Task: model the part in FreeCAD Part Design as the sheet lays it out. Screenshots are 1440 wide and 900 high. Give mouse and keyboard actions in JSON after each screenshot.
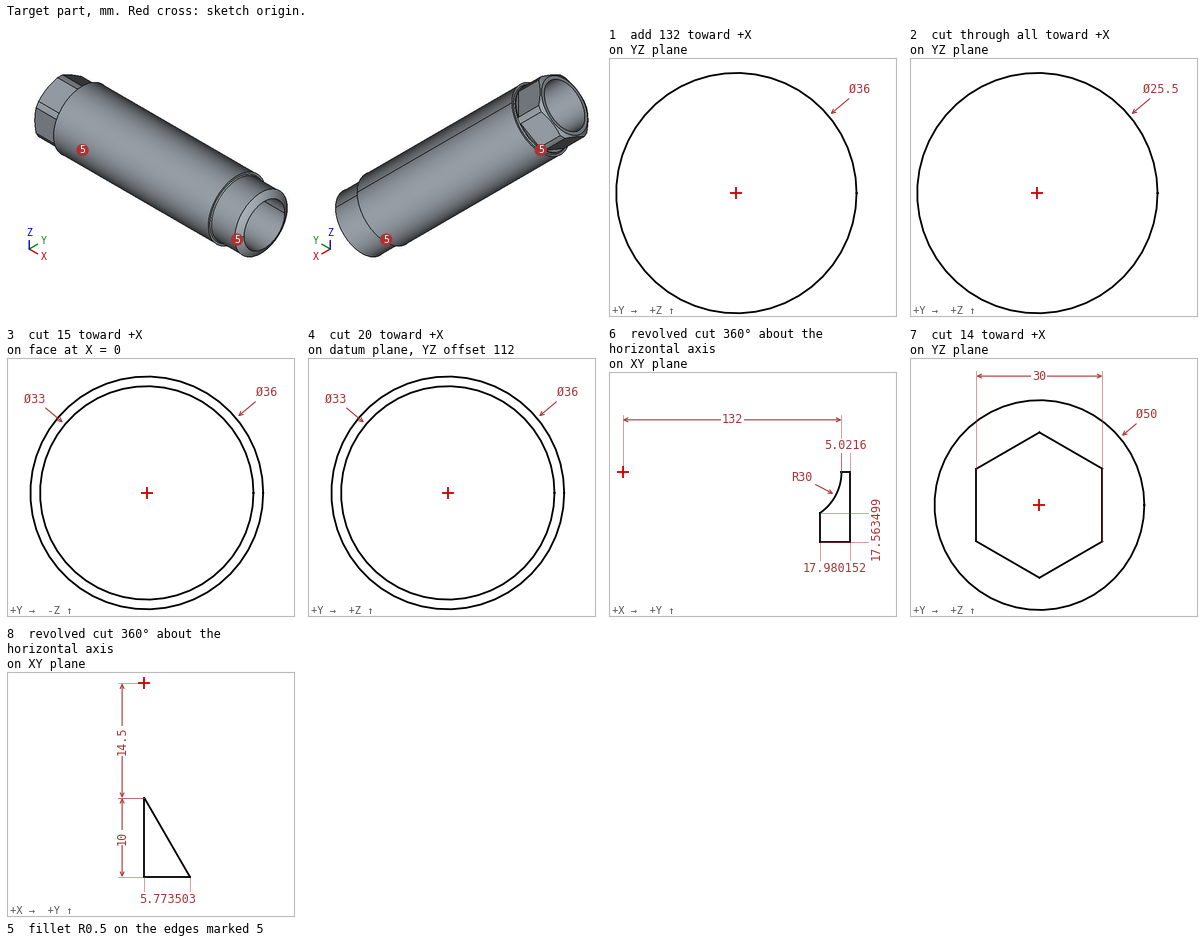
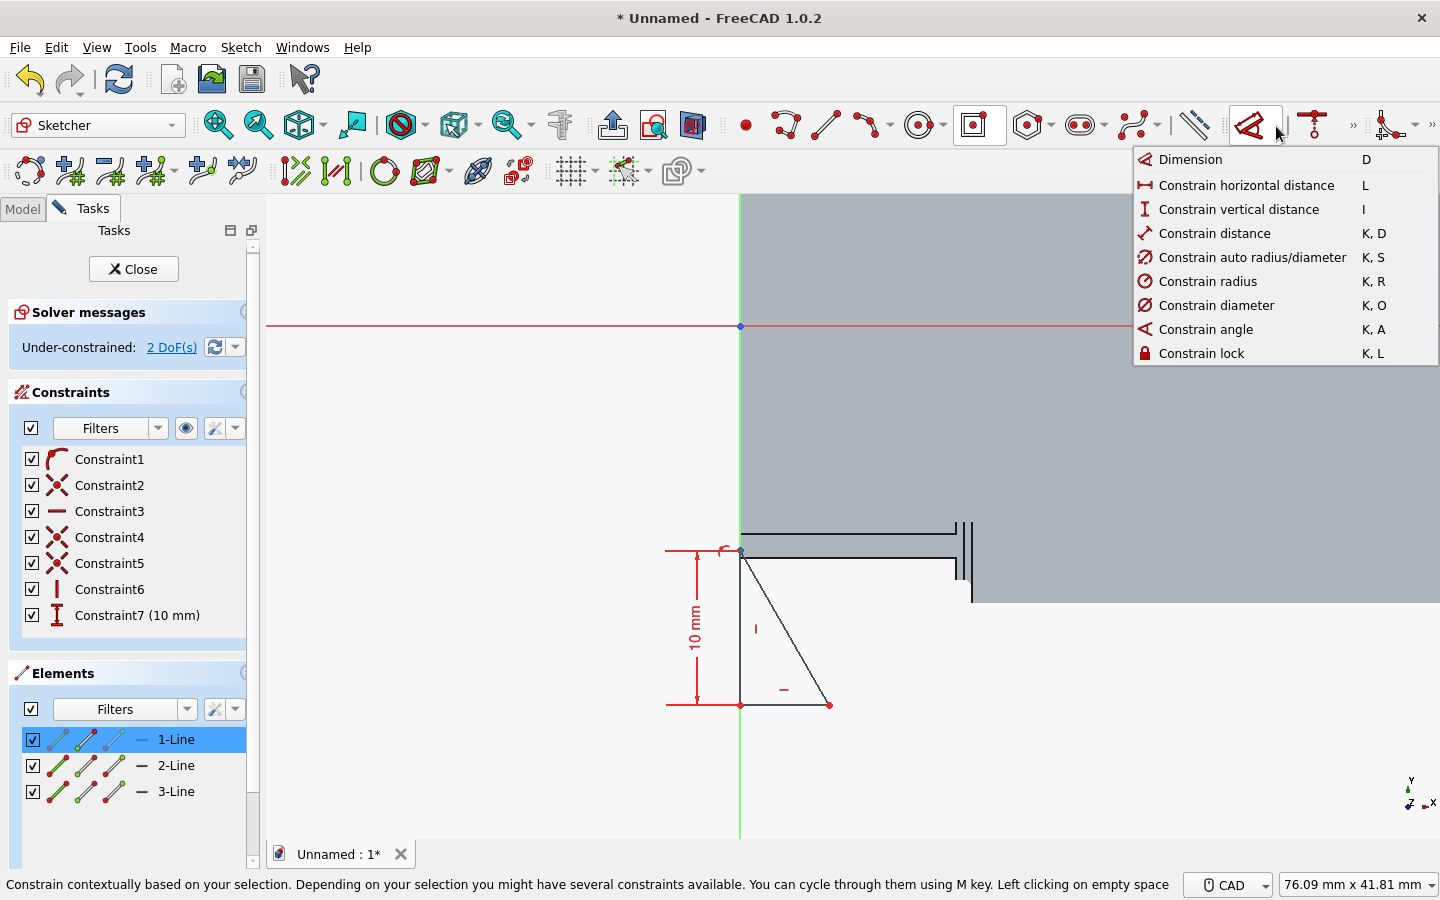
{"action": "left_click", "coordinate": [1286, 209]}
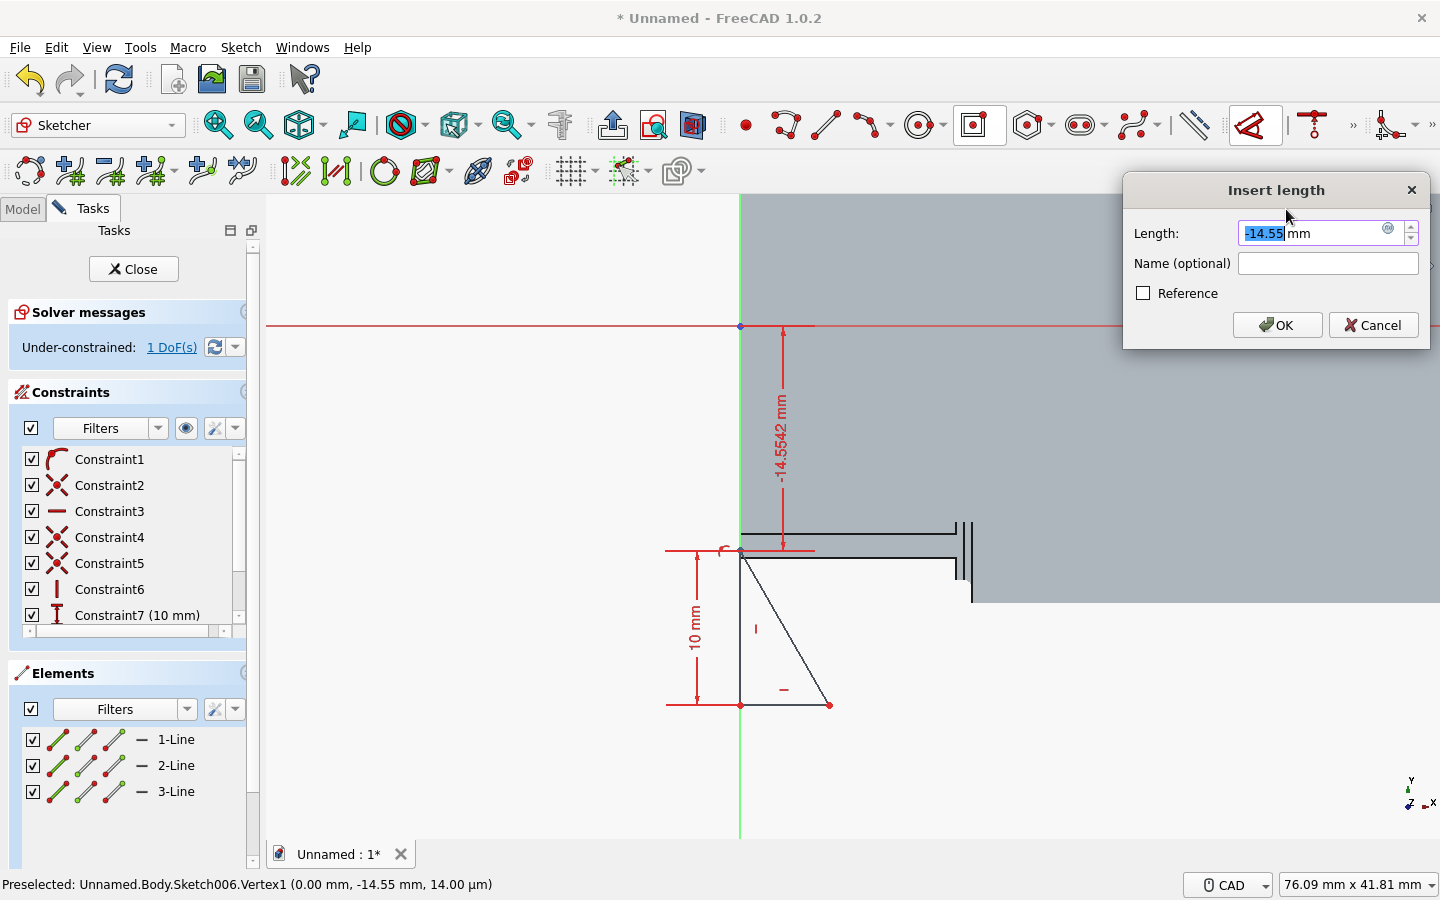
{"action": "type", "text": "-14.5"}
{"action": "key", "text": "Return"}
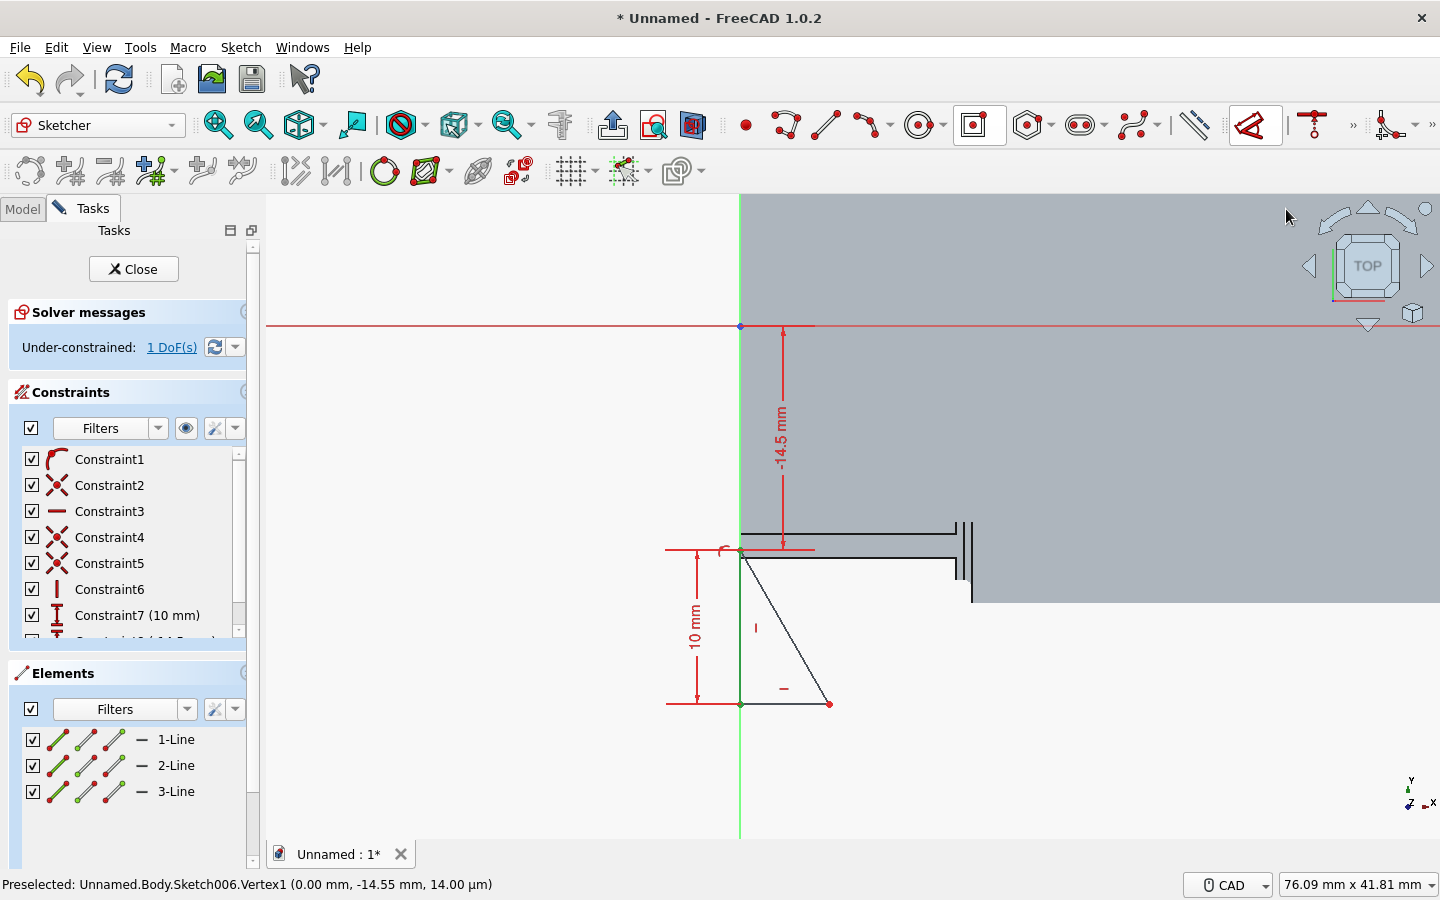
{"action": "left_click", "coordinate": [767, 704]}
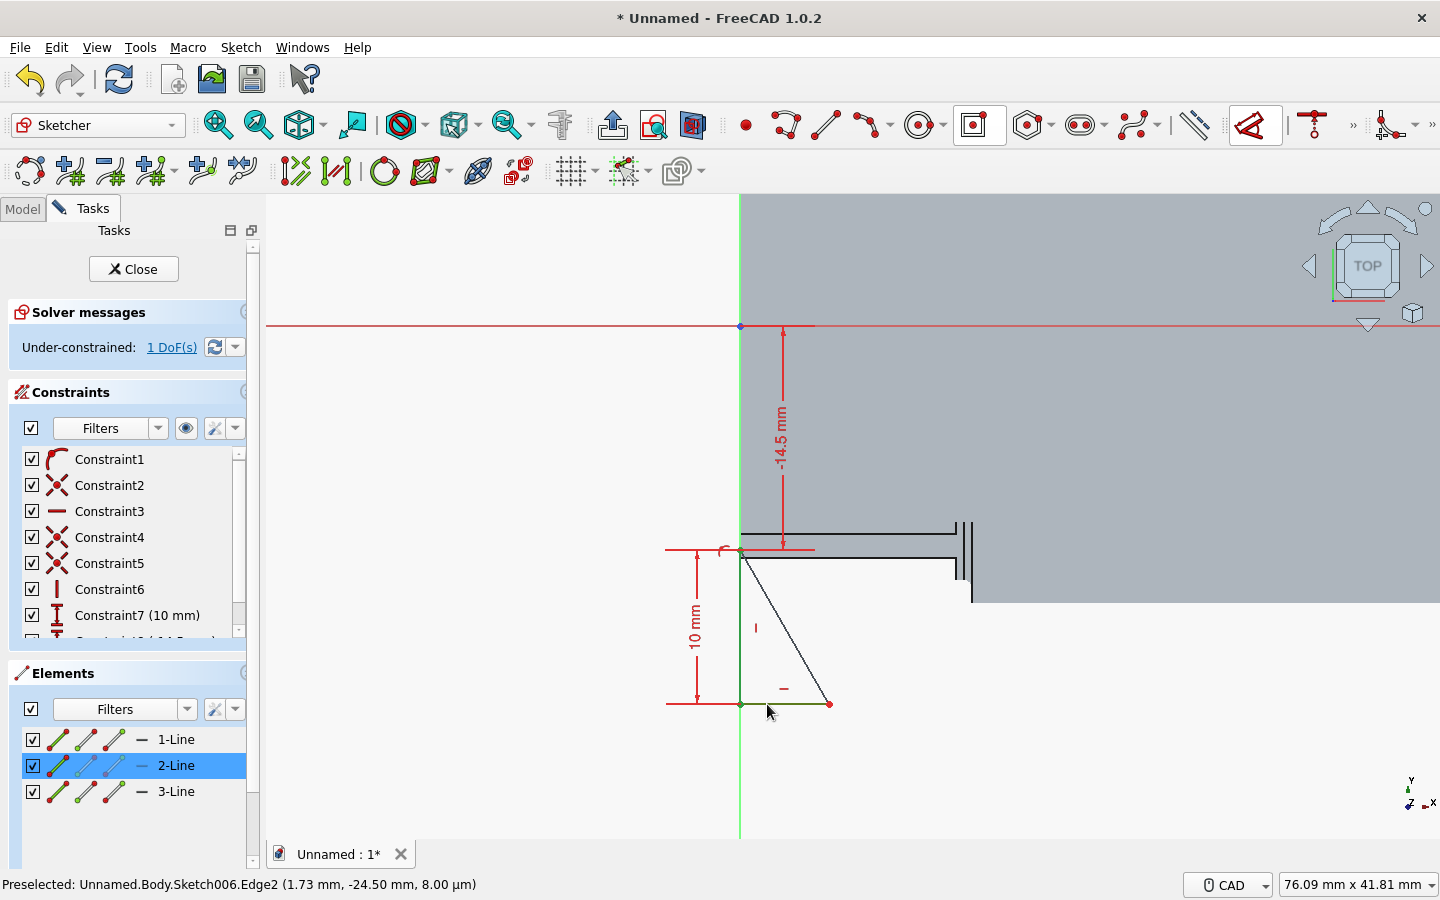
{"action": "key", "text": "l"}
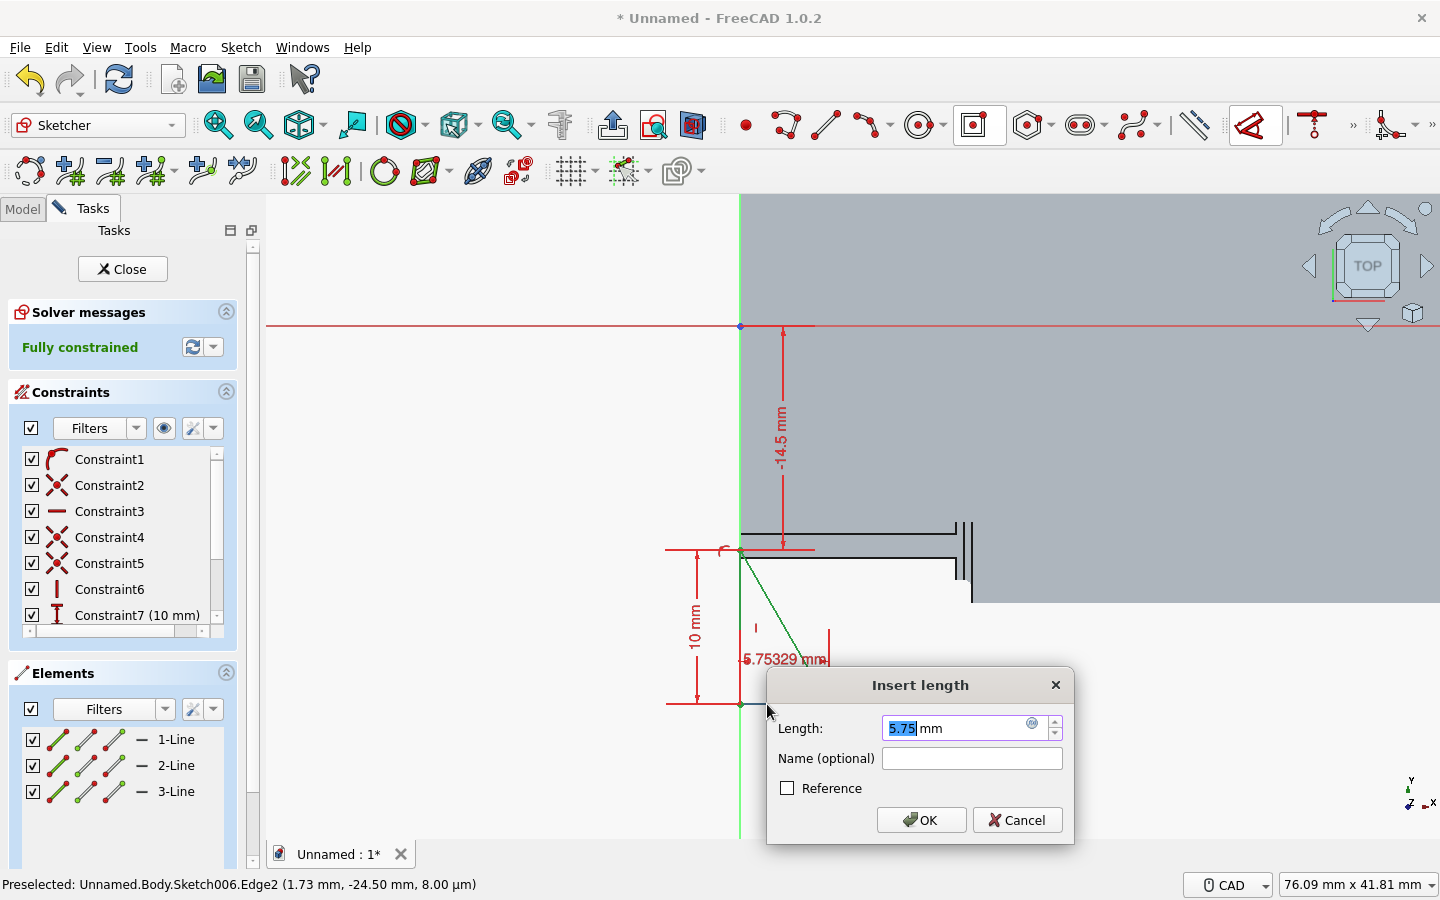
{"action": "type", "text": "5.773503"}
{"action": "key", "text": "Return"}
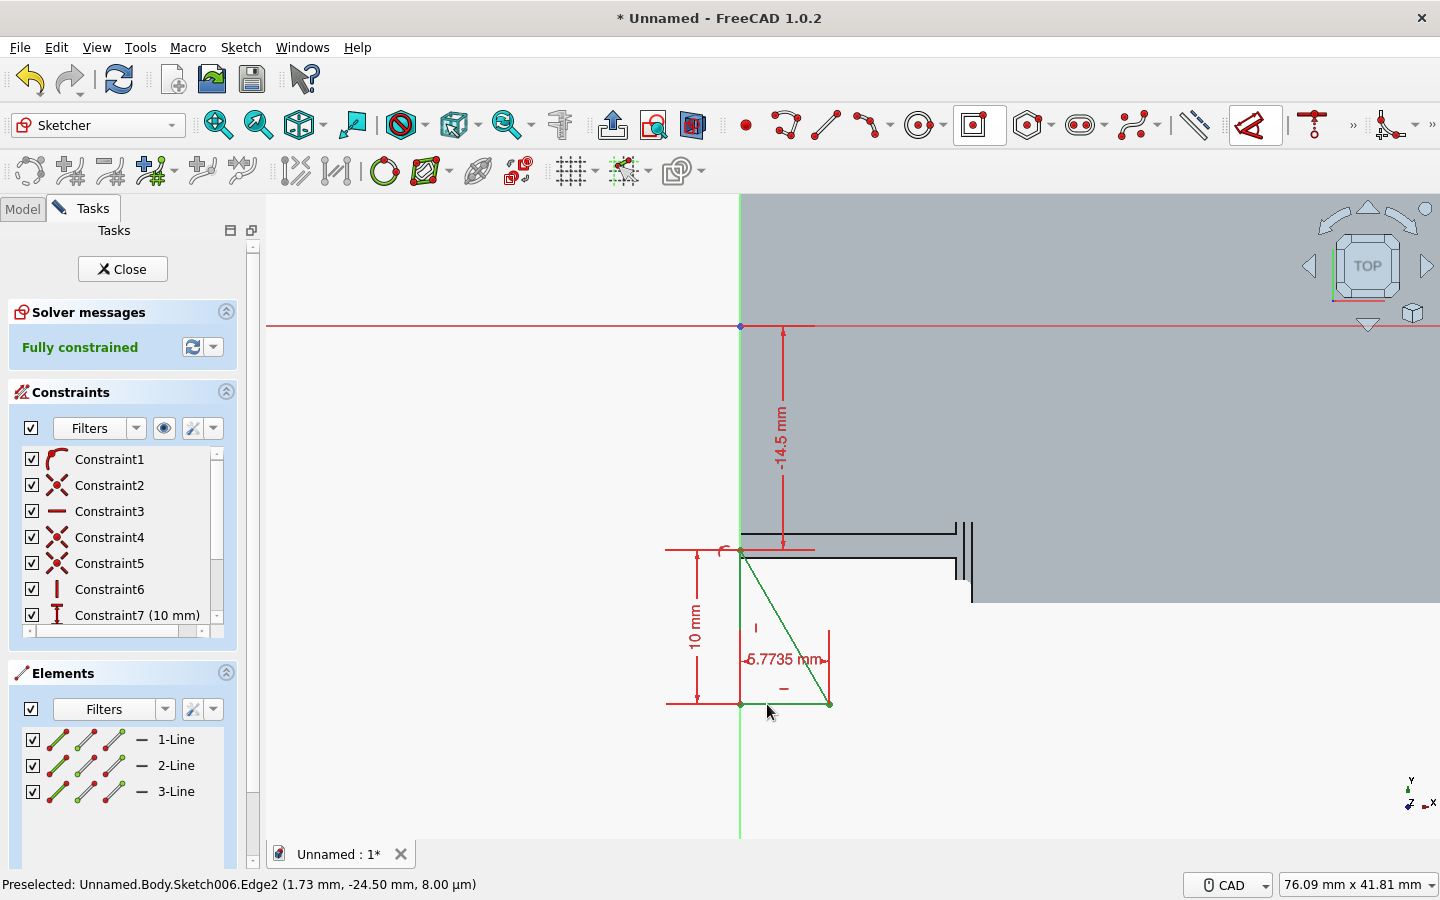
{"action": "left_click", "coordinate": [123, 269]}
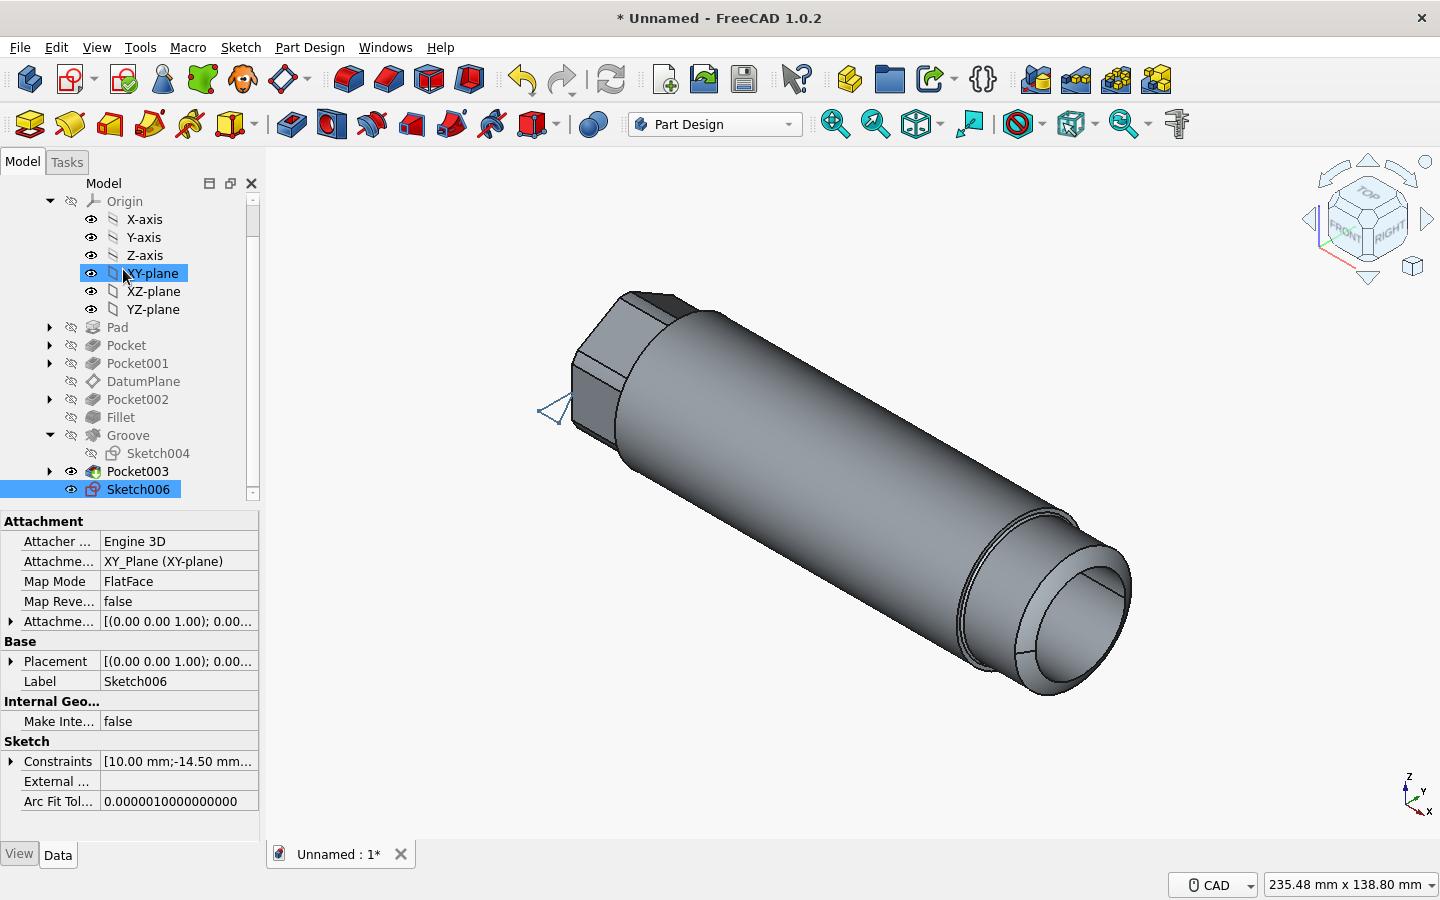
{"action": "left_click", "coordinate": [372, 124]}